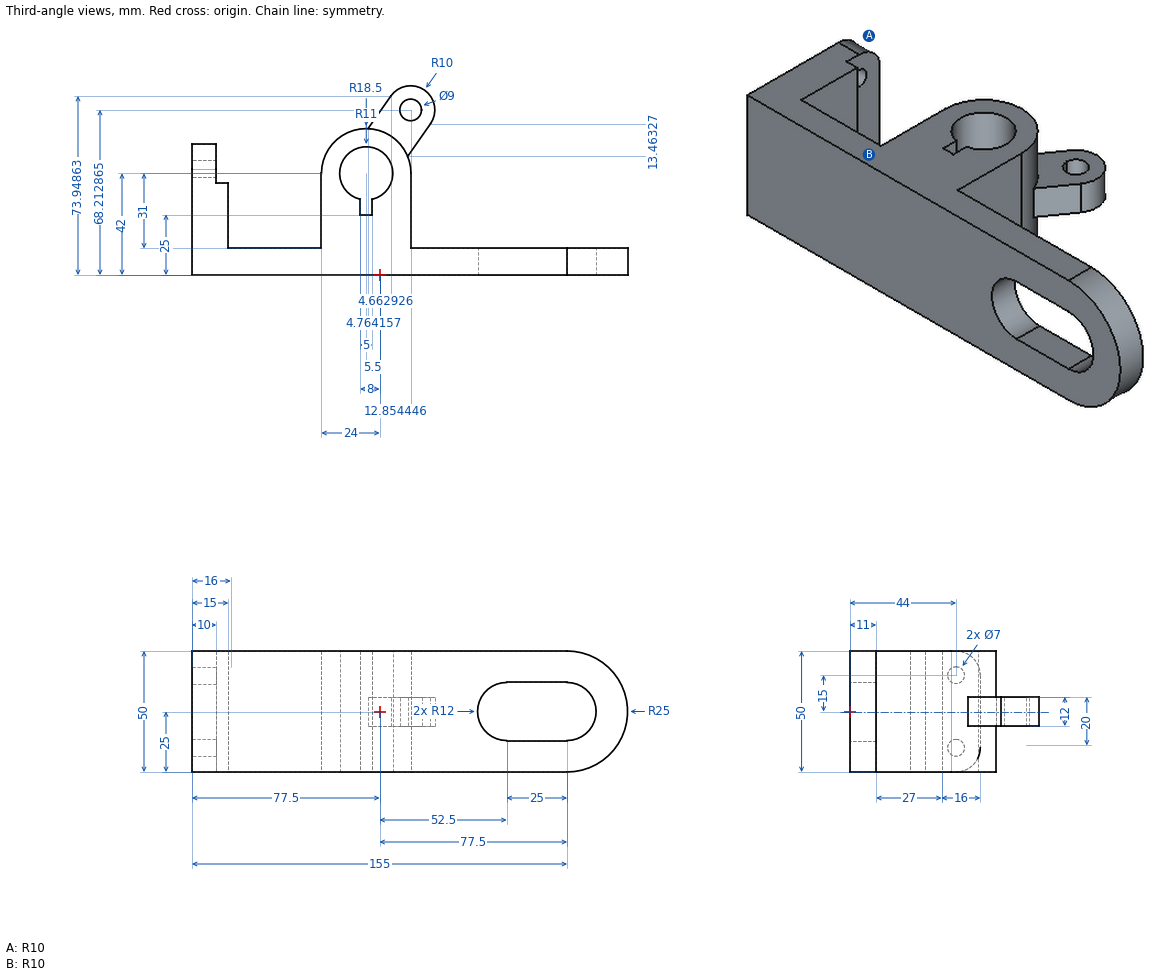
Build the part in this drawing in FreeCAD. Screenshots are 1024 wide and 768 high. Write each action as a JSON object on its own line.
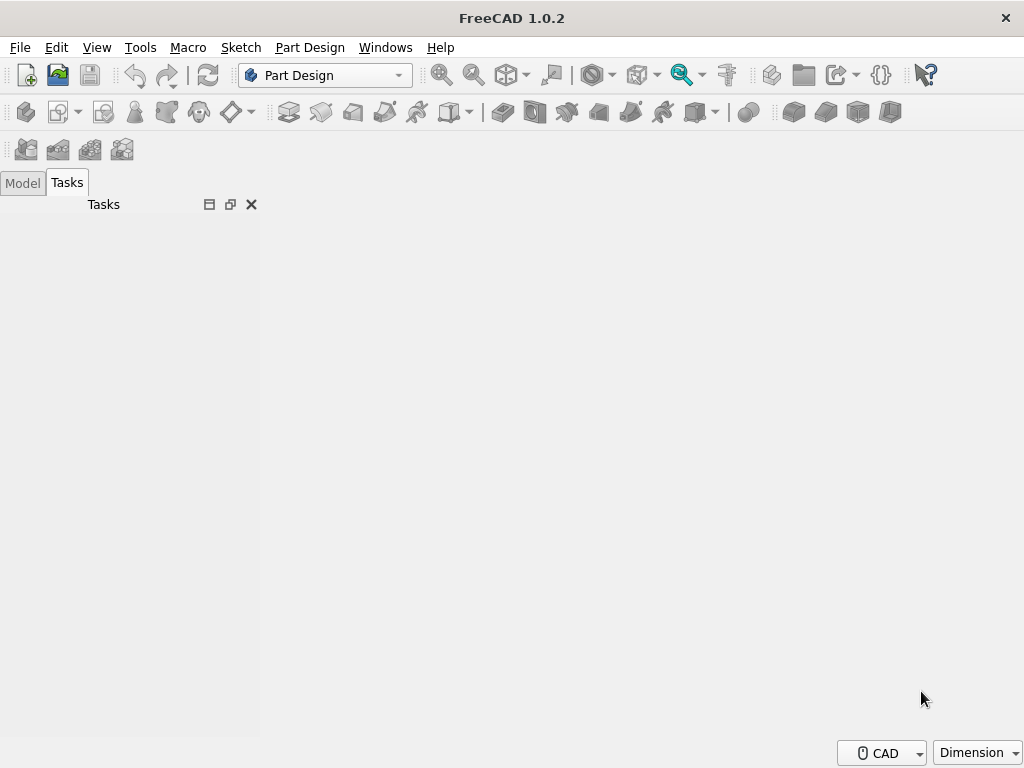
{"action": "left_click", "coordinate": [26, 76]}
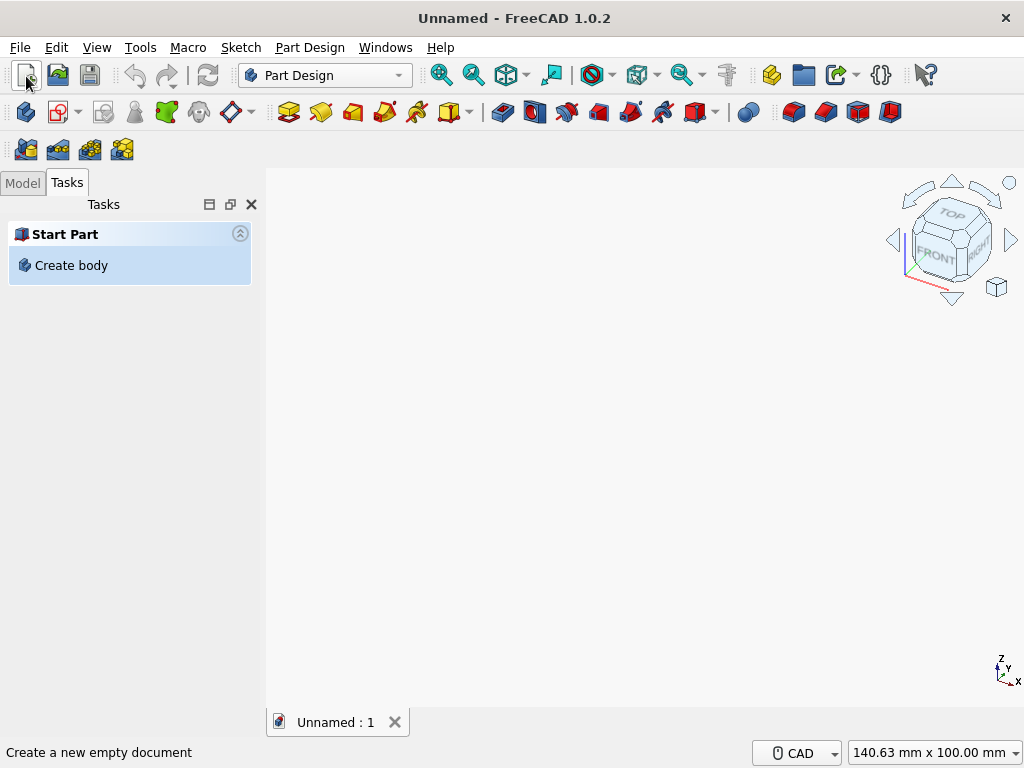
{"action": "left_click", "coordinate": [58, 112]}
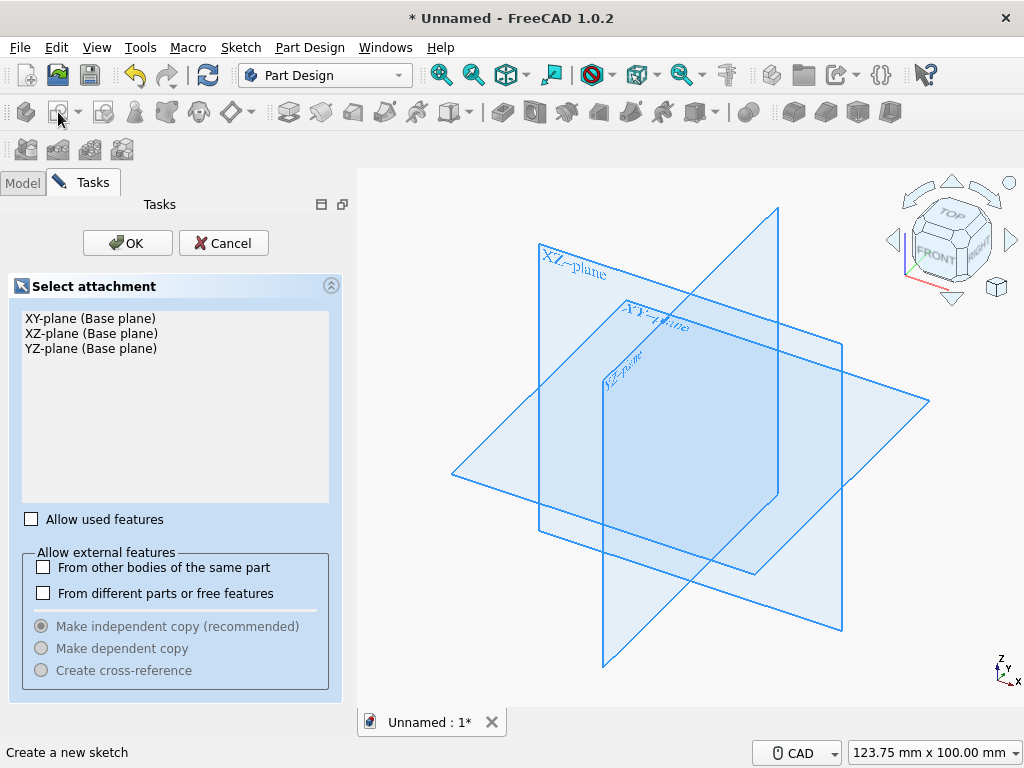
{"action": "left_click", "coordinate": [82, 334]}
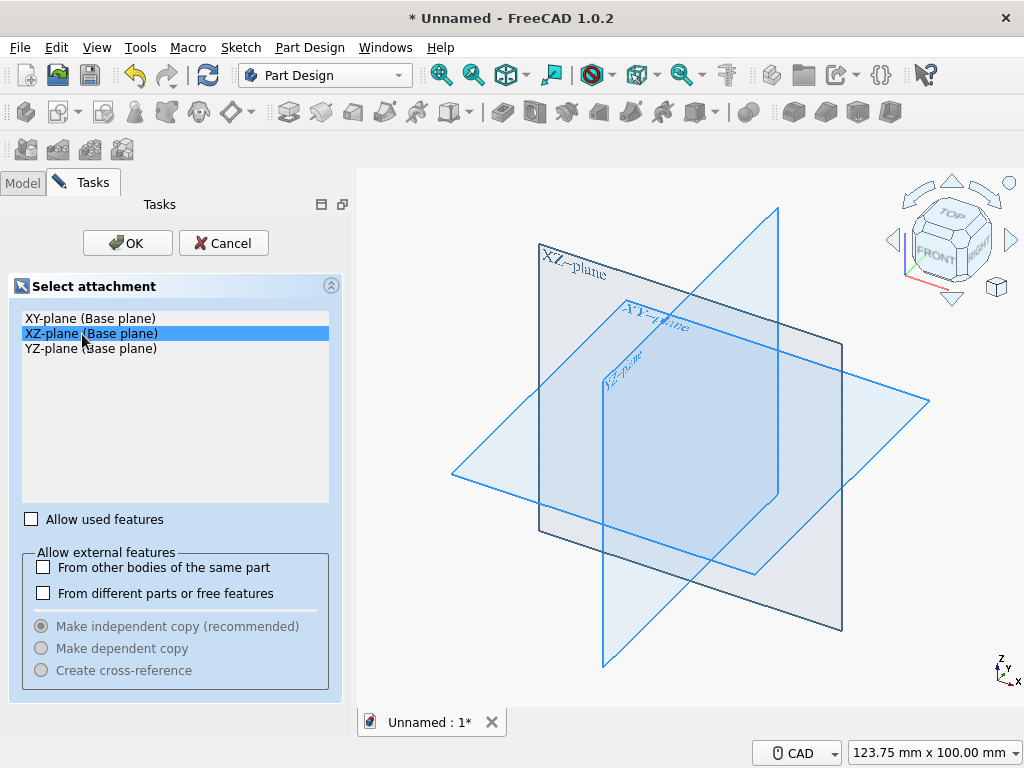
{"action": "left_click", "coordinate": [128, 243]}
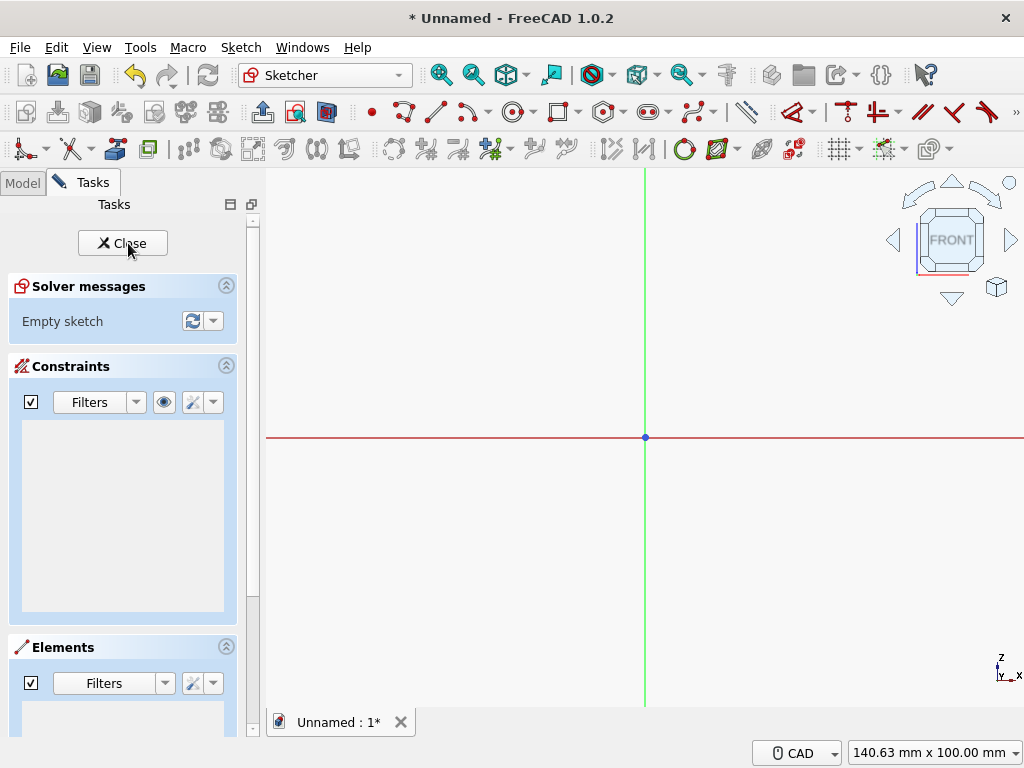
{"action": "scroll", "coordinate": [466, 438], "scroll_direction": "down", "scroll_amount": 4}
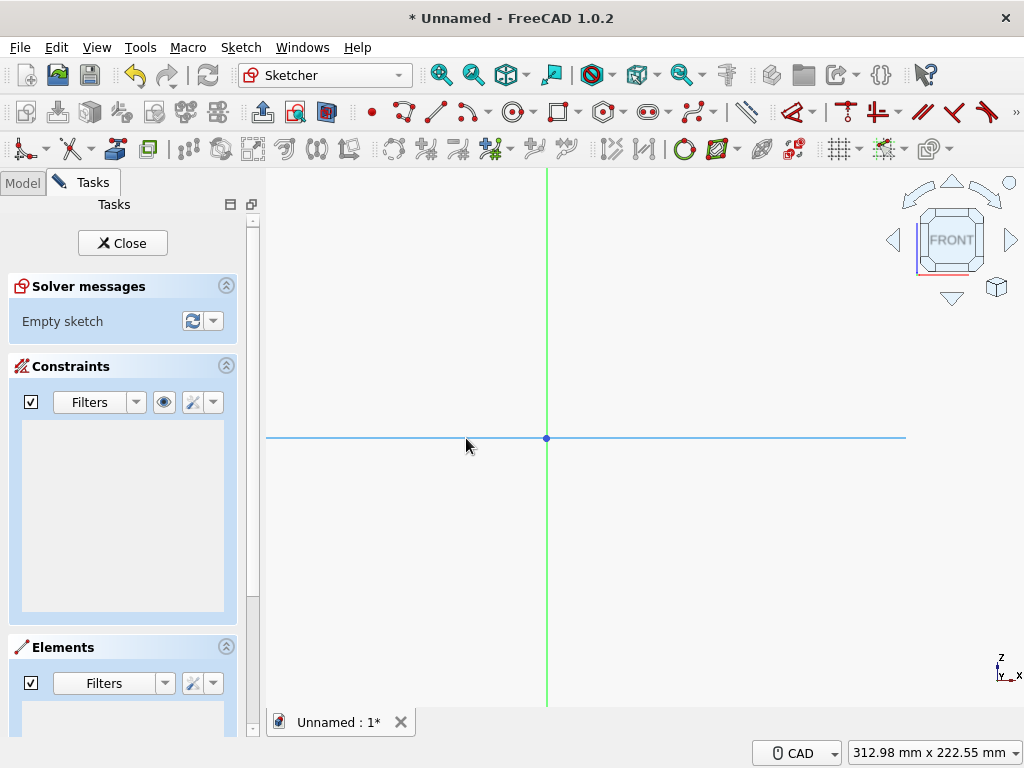
{"action": "left_click", "coordinate": [404, 112]}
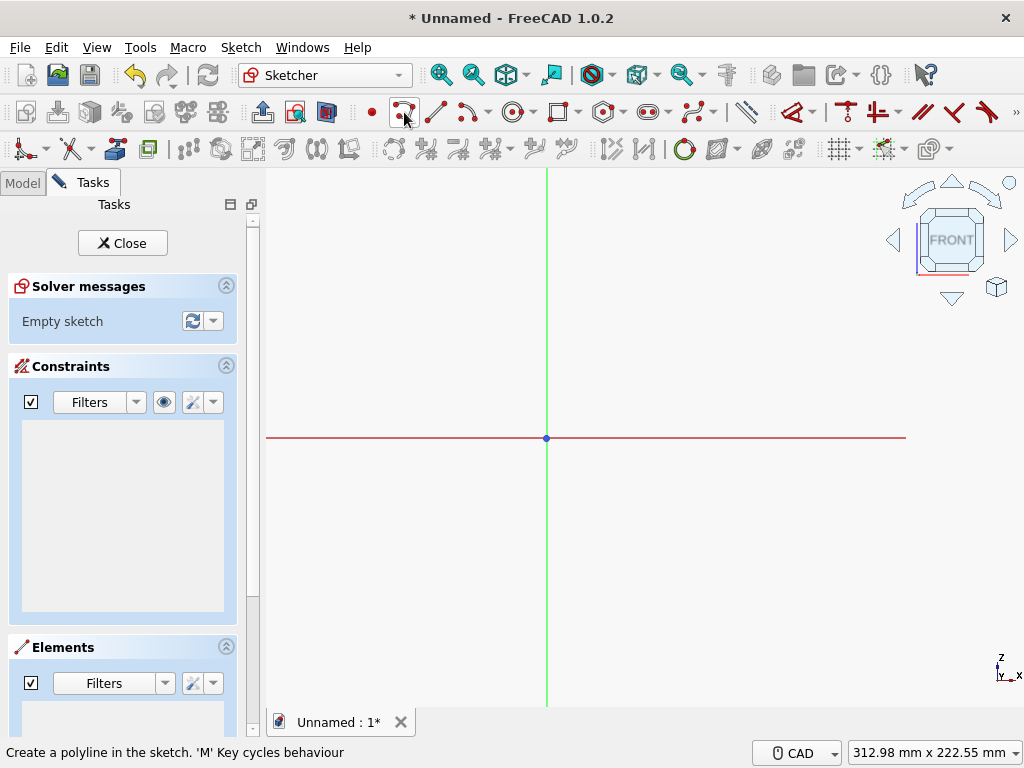
{"action": "left_click", "coordinate": [734, 499]}
{"action": "left_click", "coordinate": [359, 499]}
{"action": "left_click", "coordinate": [359, 378]}
{"action": "left_click", "coordinate": [734, 378]}
{"action": "right_click", "coordinate": [734, 378]}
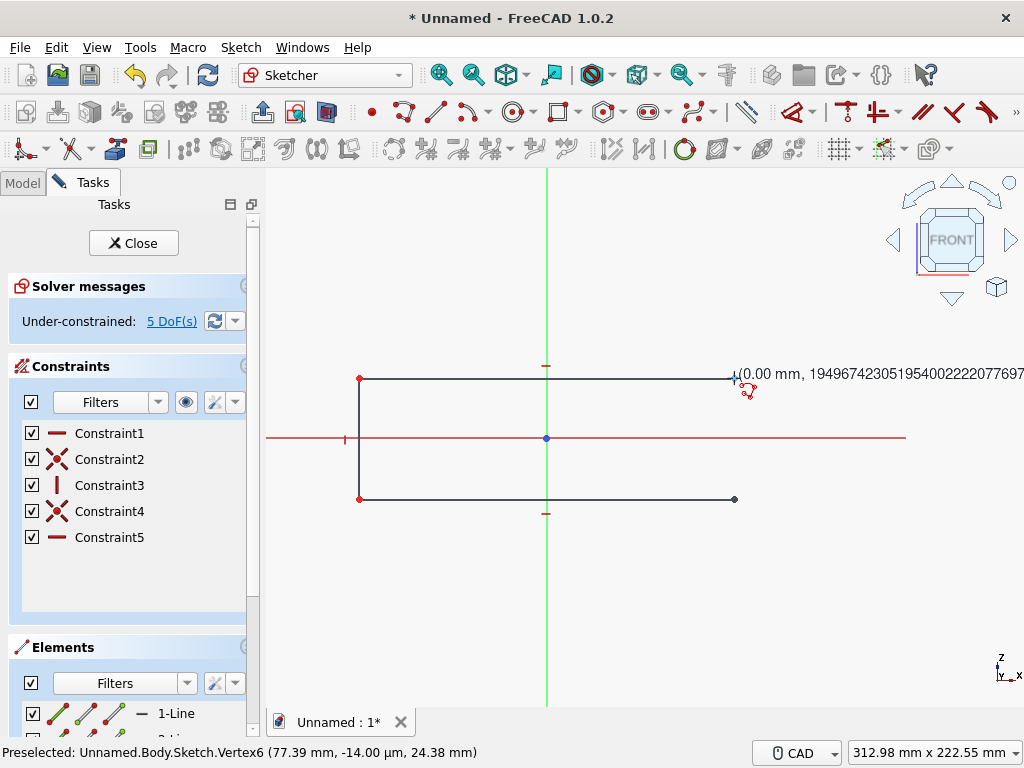
{"action": "key", "text": "g 3 a"}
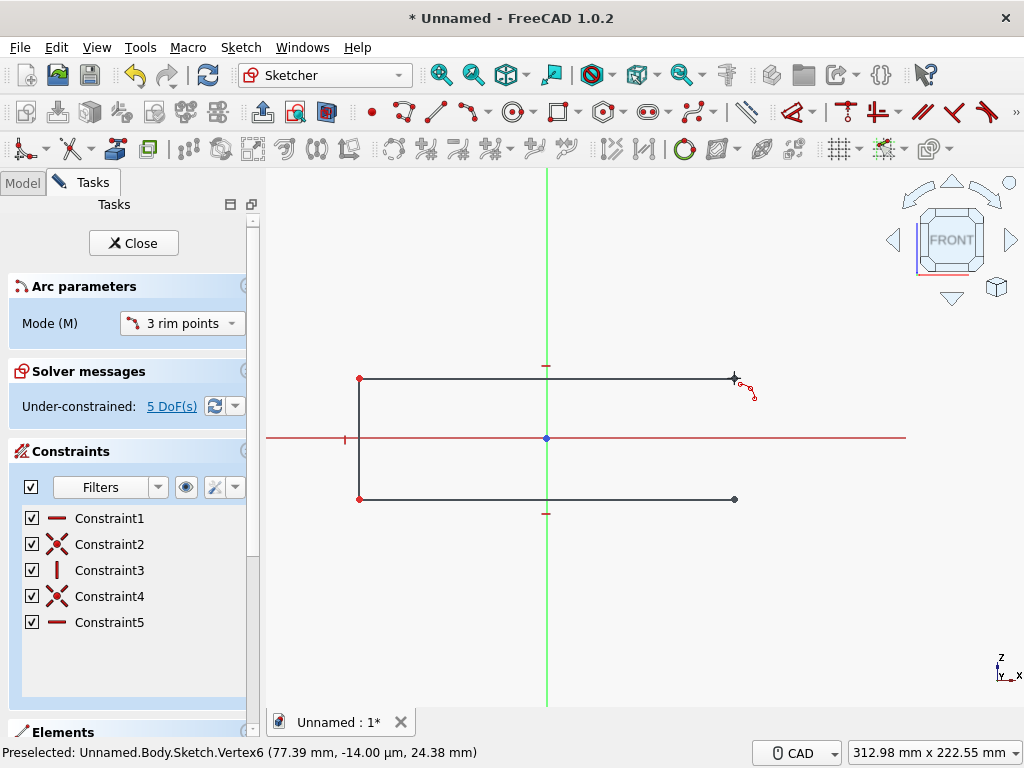
{"action": "left_click", "coordinate": [734, 379]}
{"action": "left_click", "coordinate": [734, 500]}
{"action": "left_click", "coordinate": [792, 457]}
{"action": "key", "text": "Escape"}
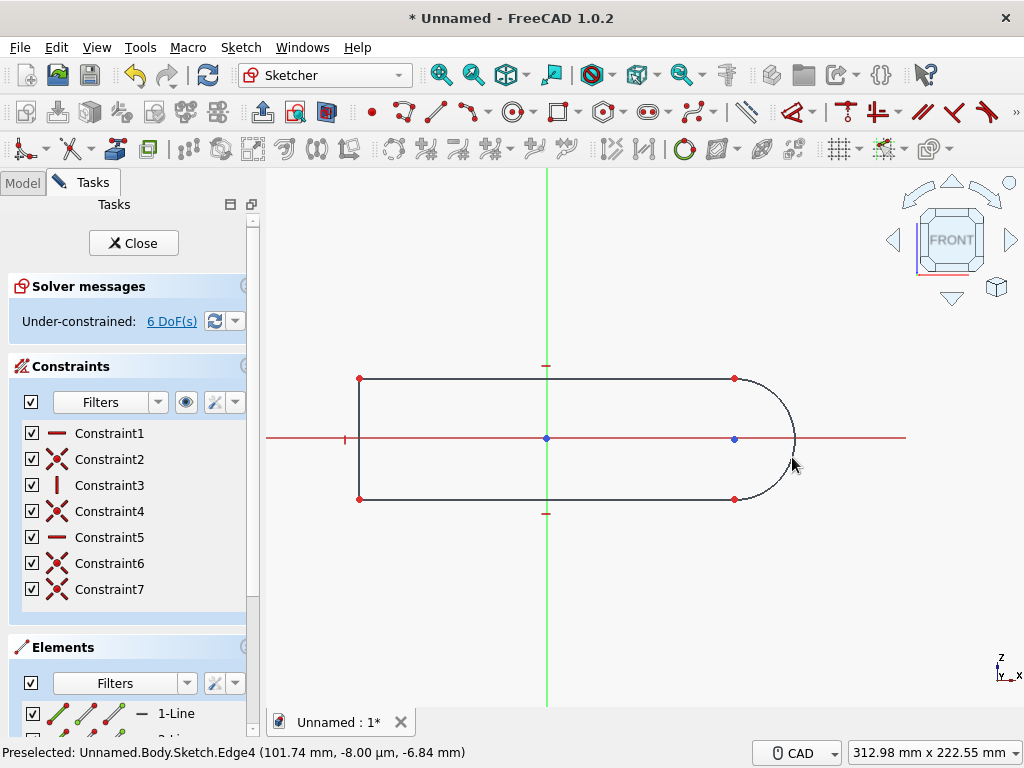
{"action": "left_click", "coordinate": [622, 500]}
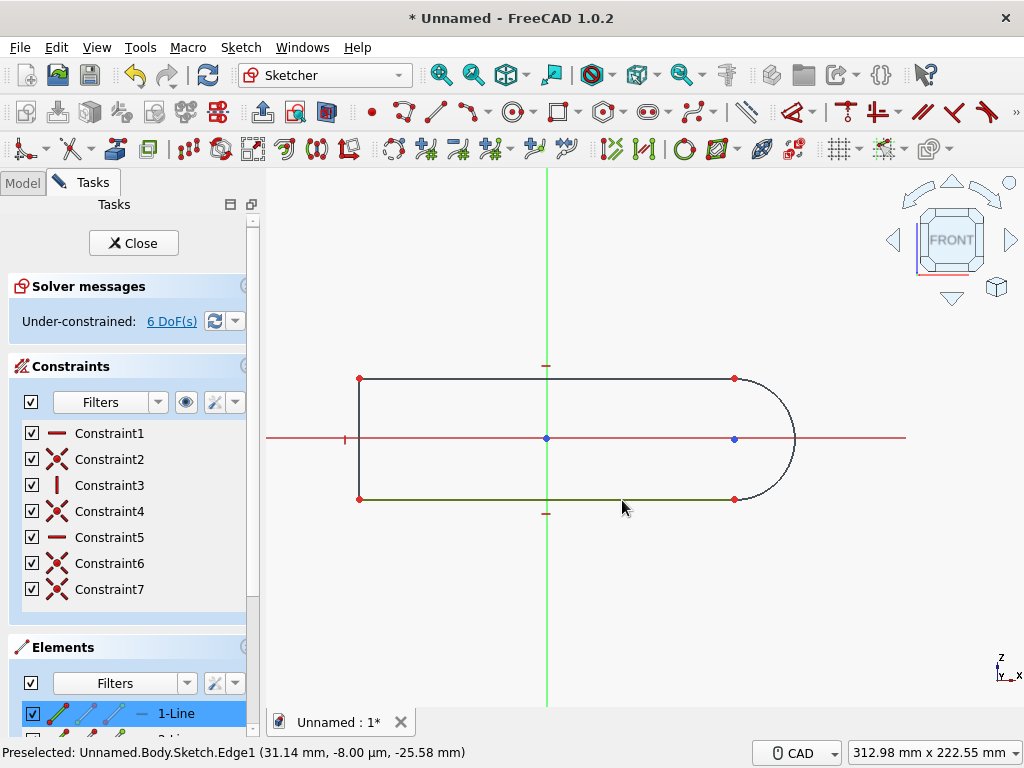
{"action": "left_click", "coordinate": [783, 475]}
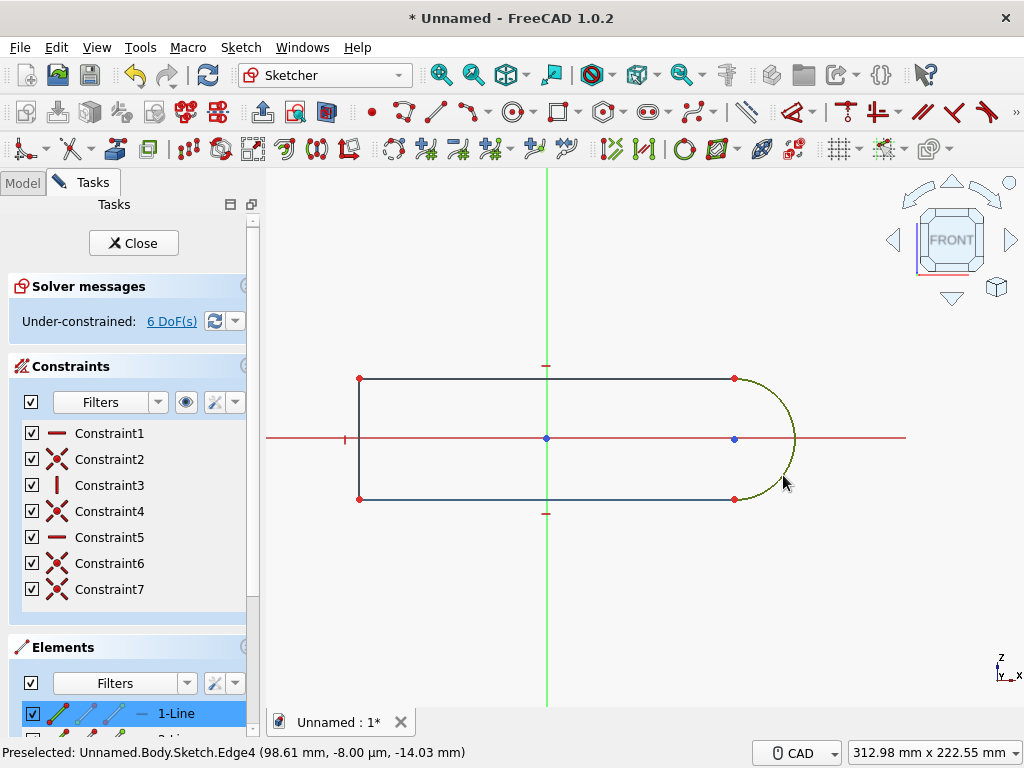
{"action": "key", "text": "t"}